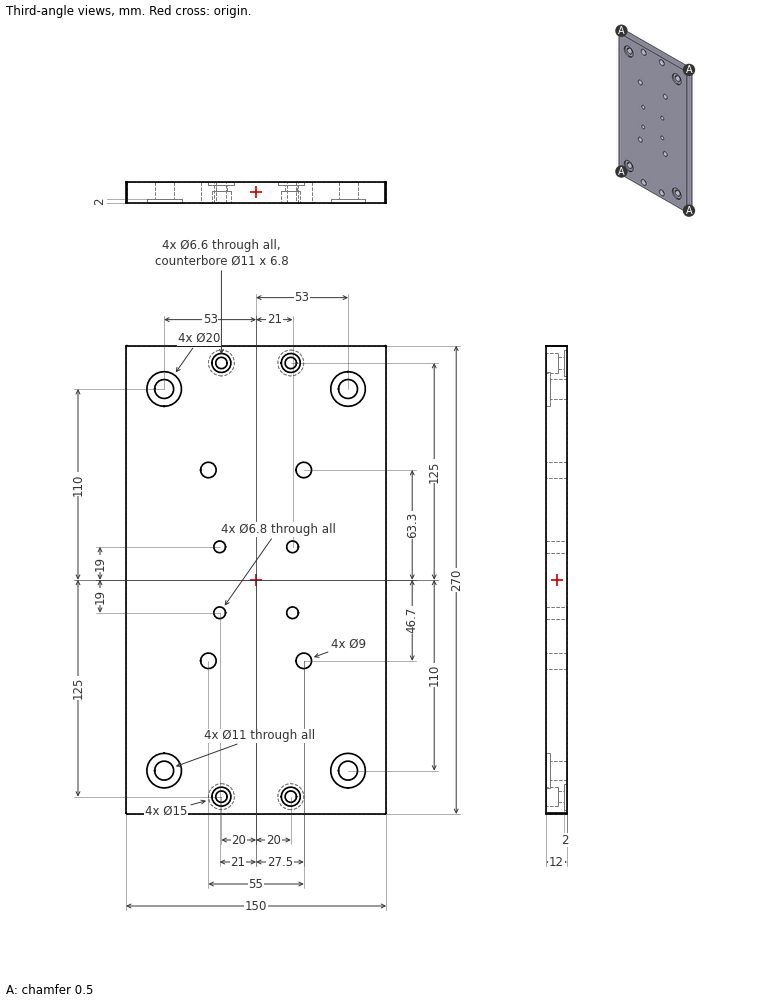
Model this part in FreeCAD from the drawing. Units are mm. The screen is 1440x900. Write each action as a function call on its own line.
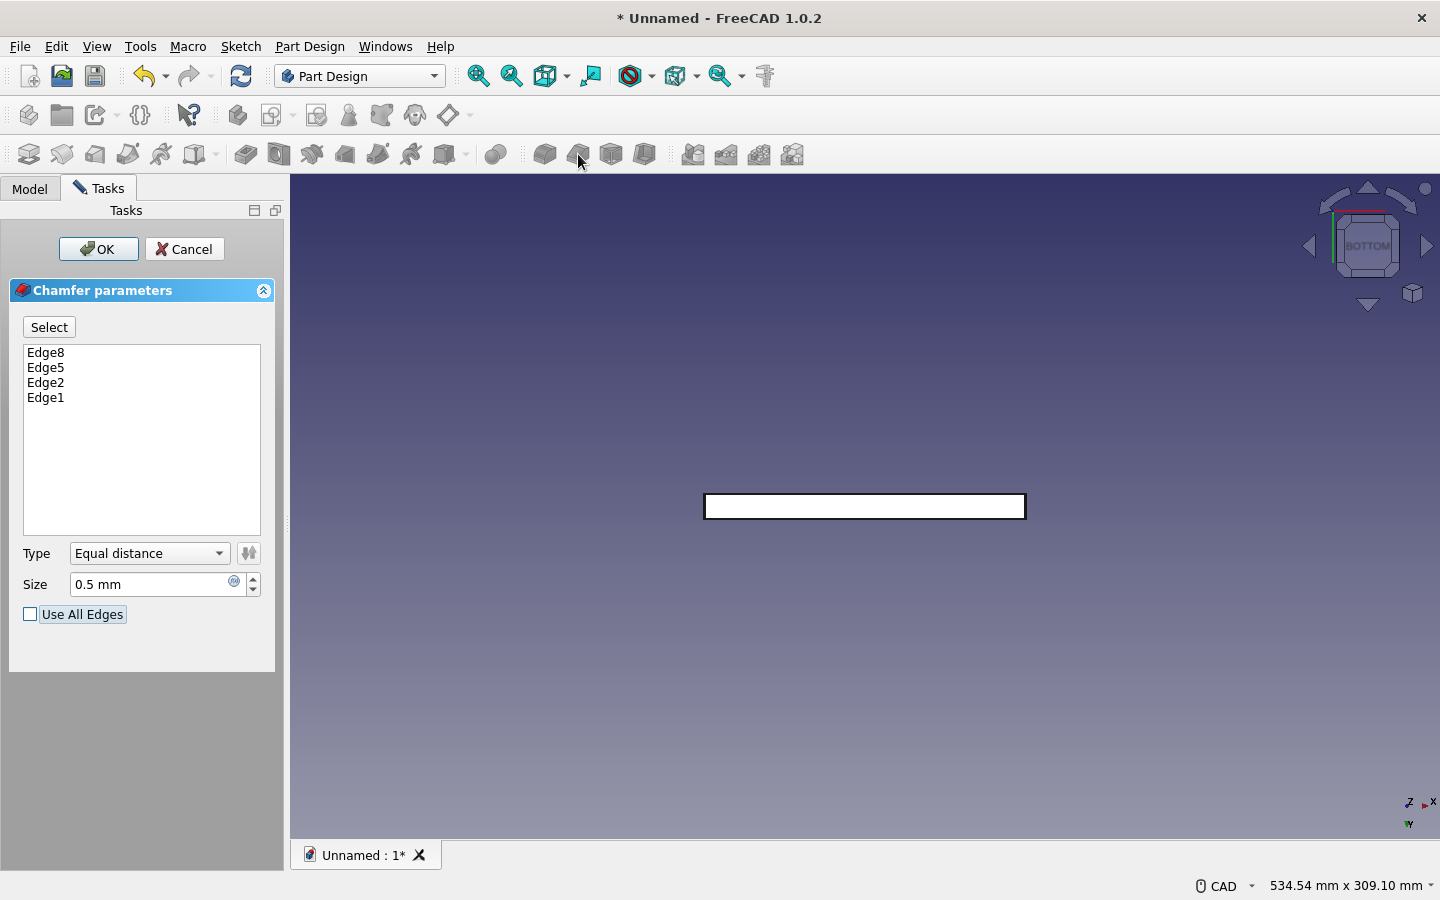
click(99, 249)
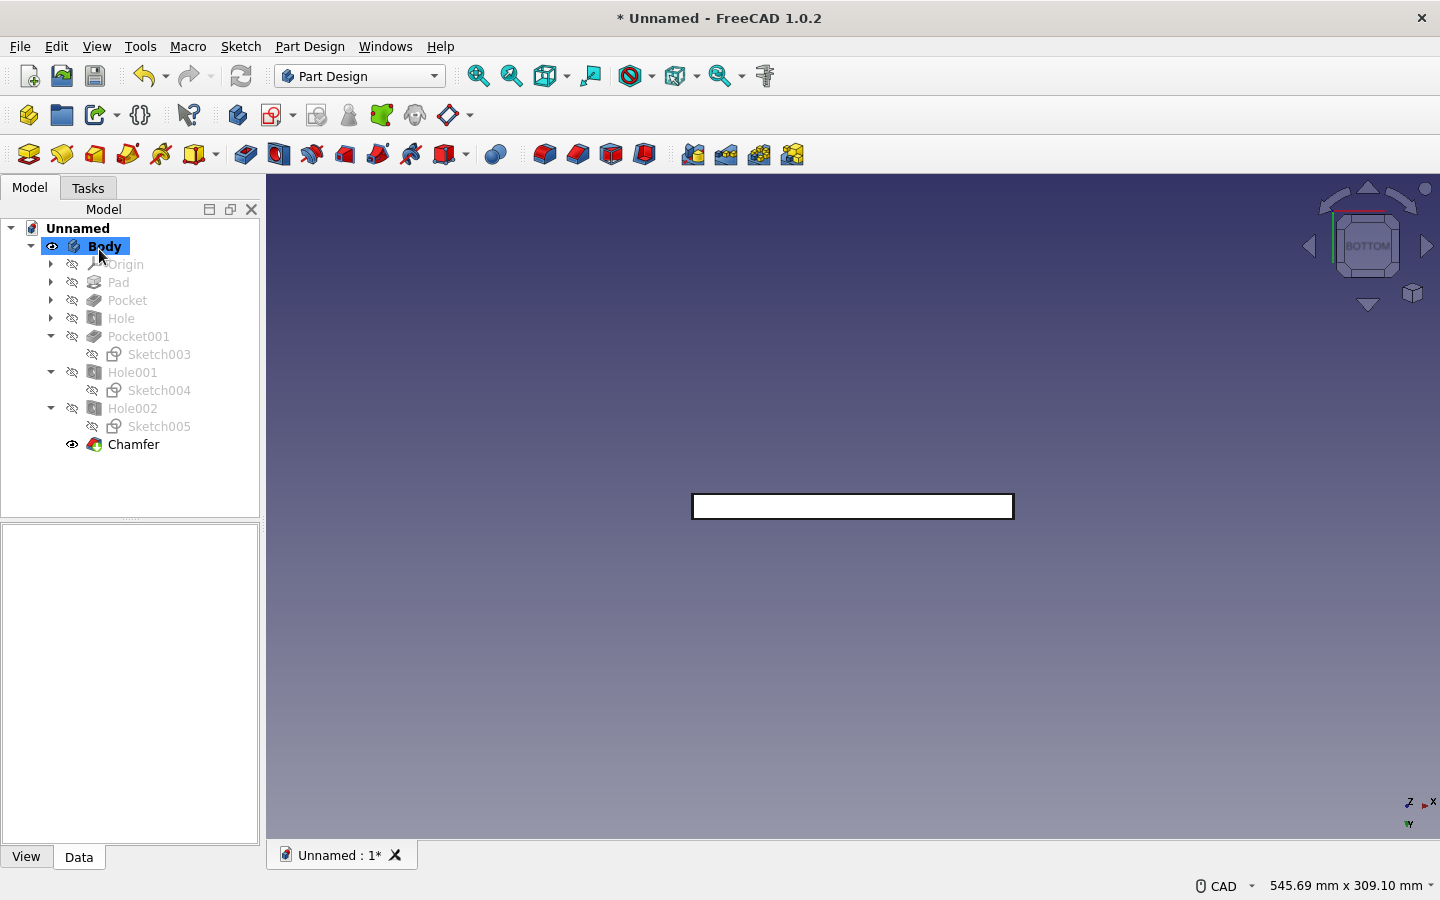
click(479, 76)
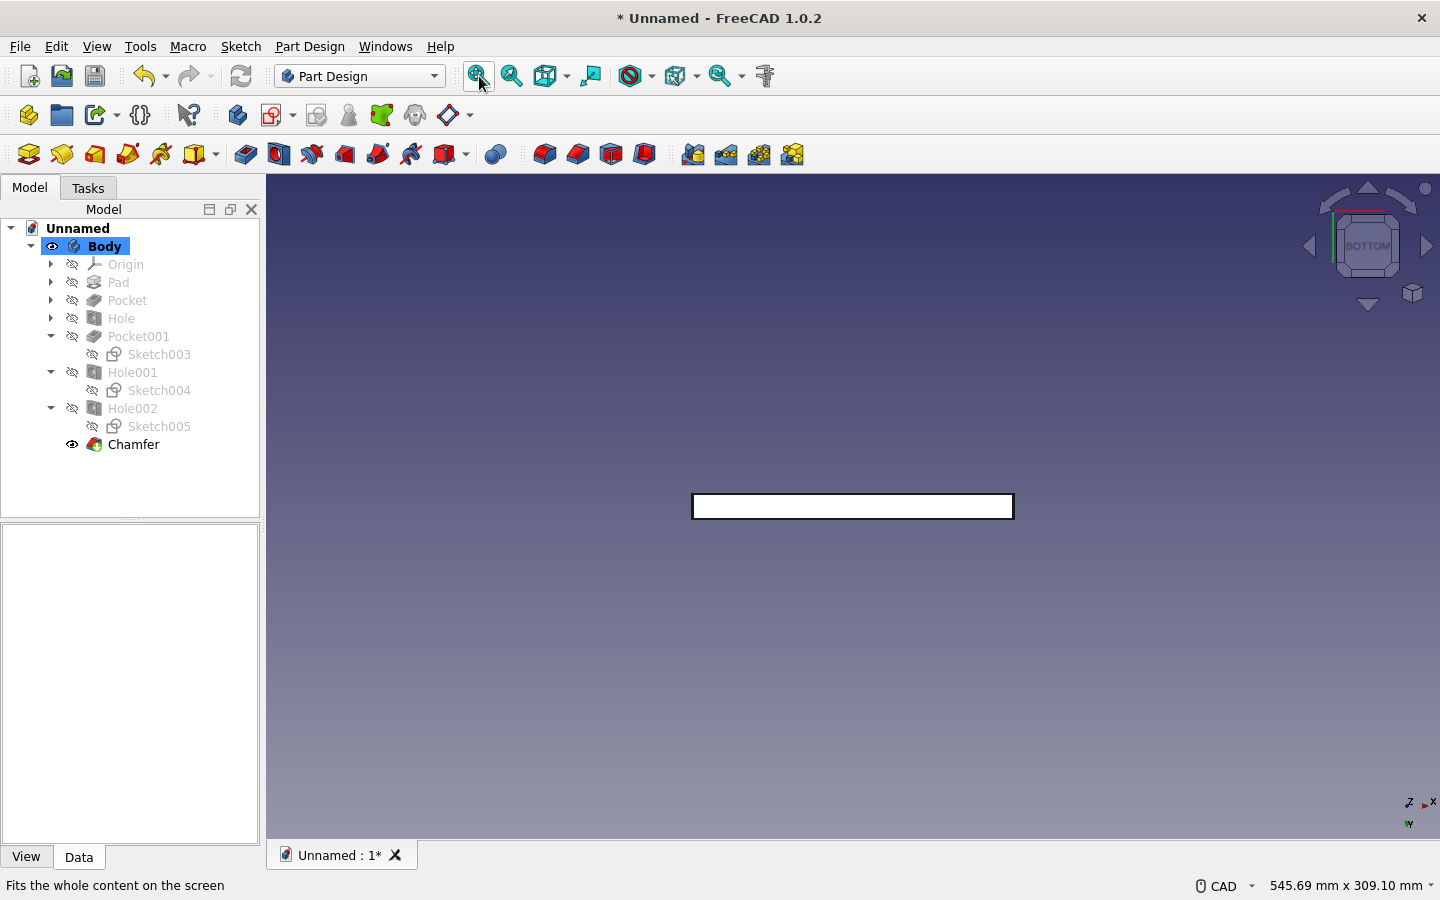
key(4)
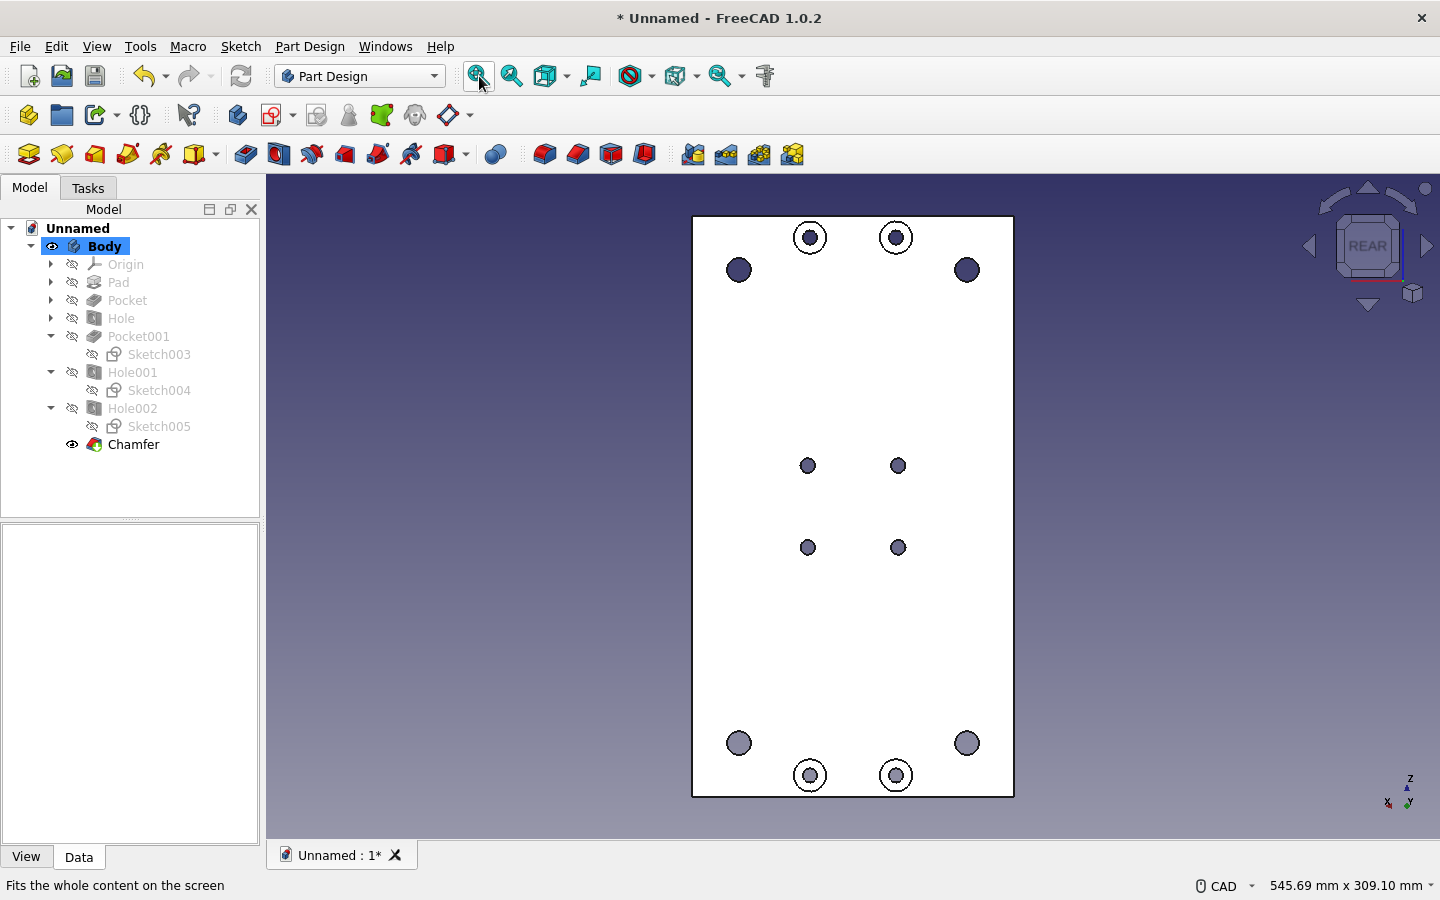
click(853, 340)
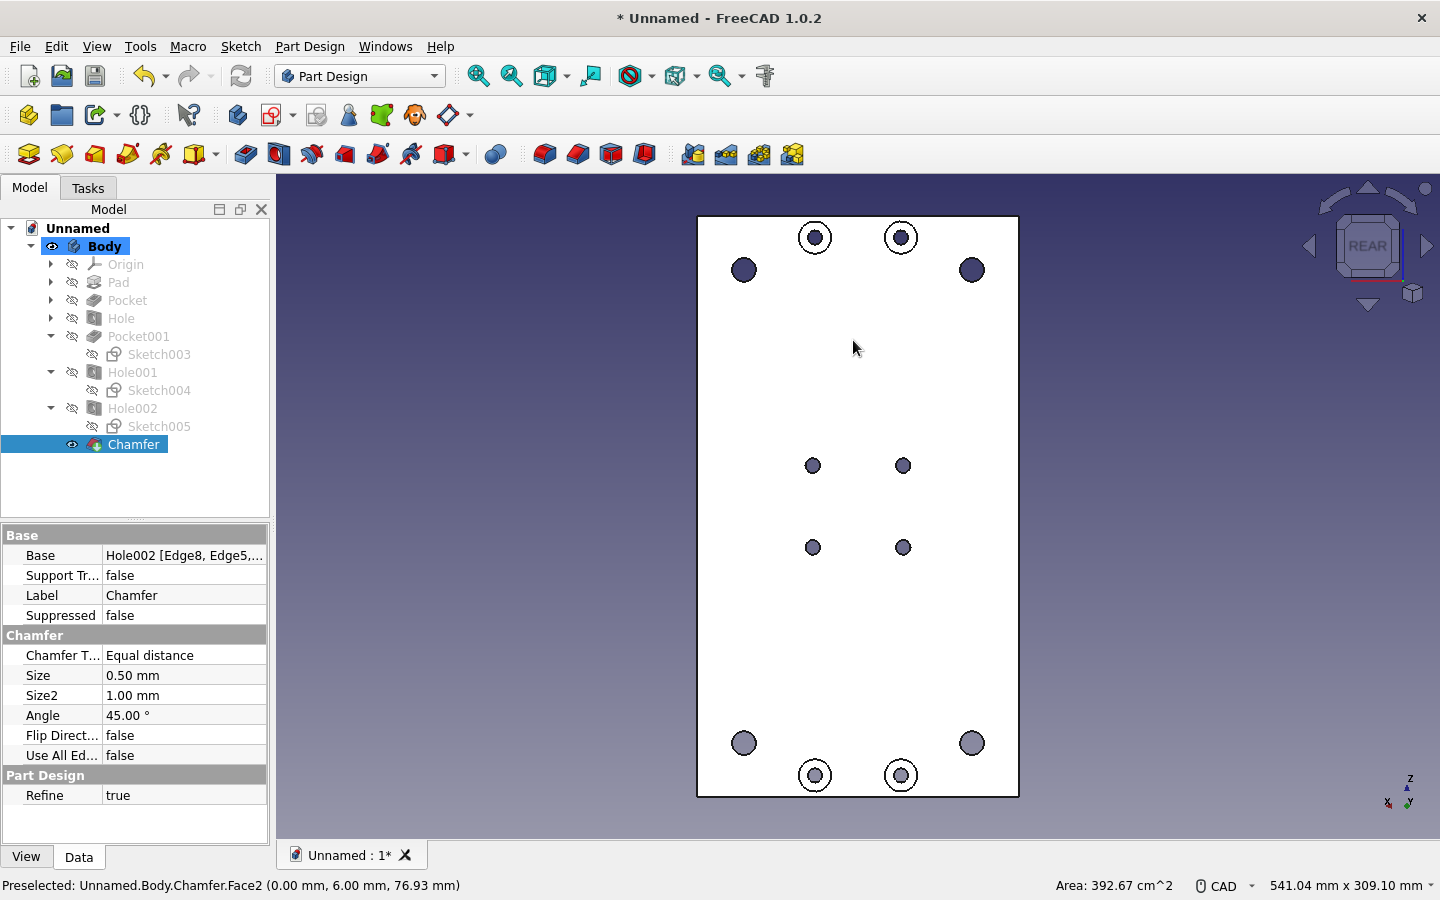
click(270, 116)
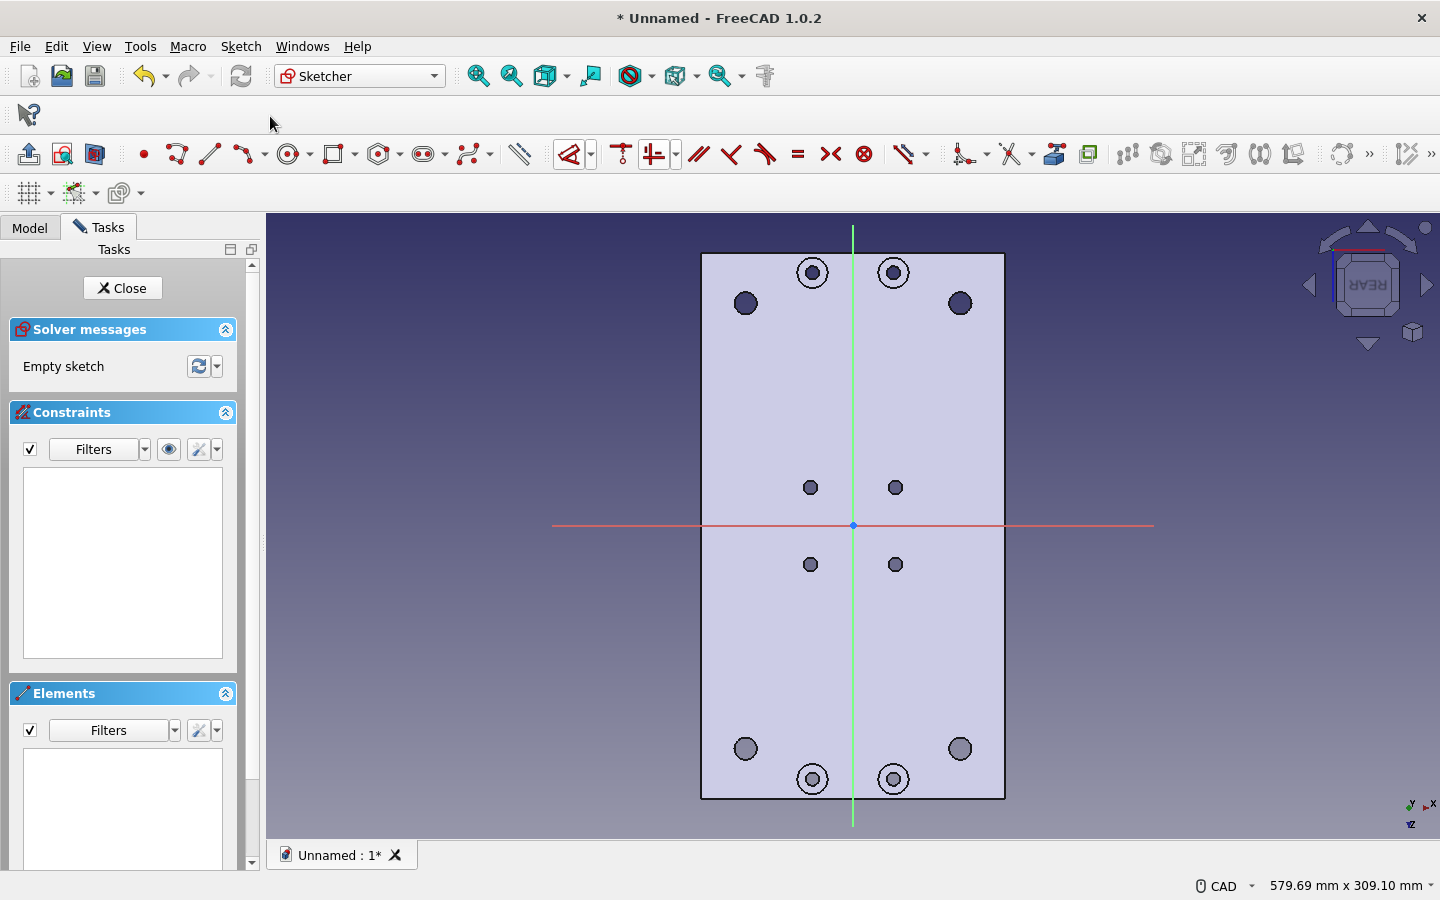
scroll(936, 563, up, 3)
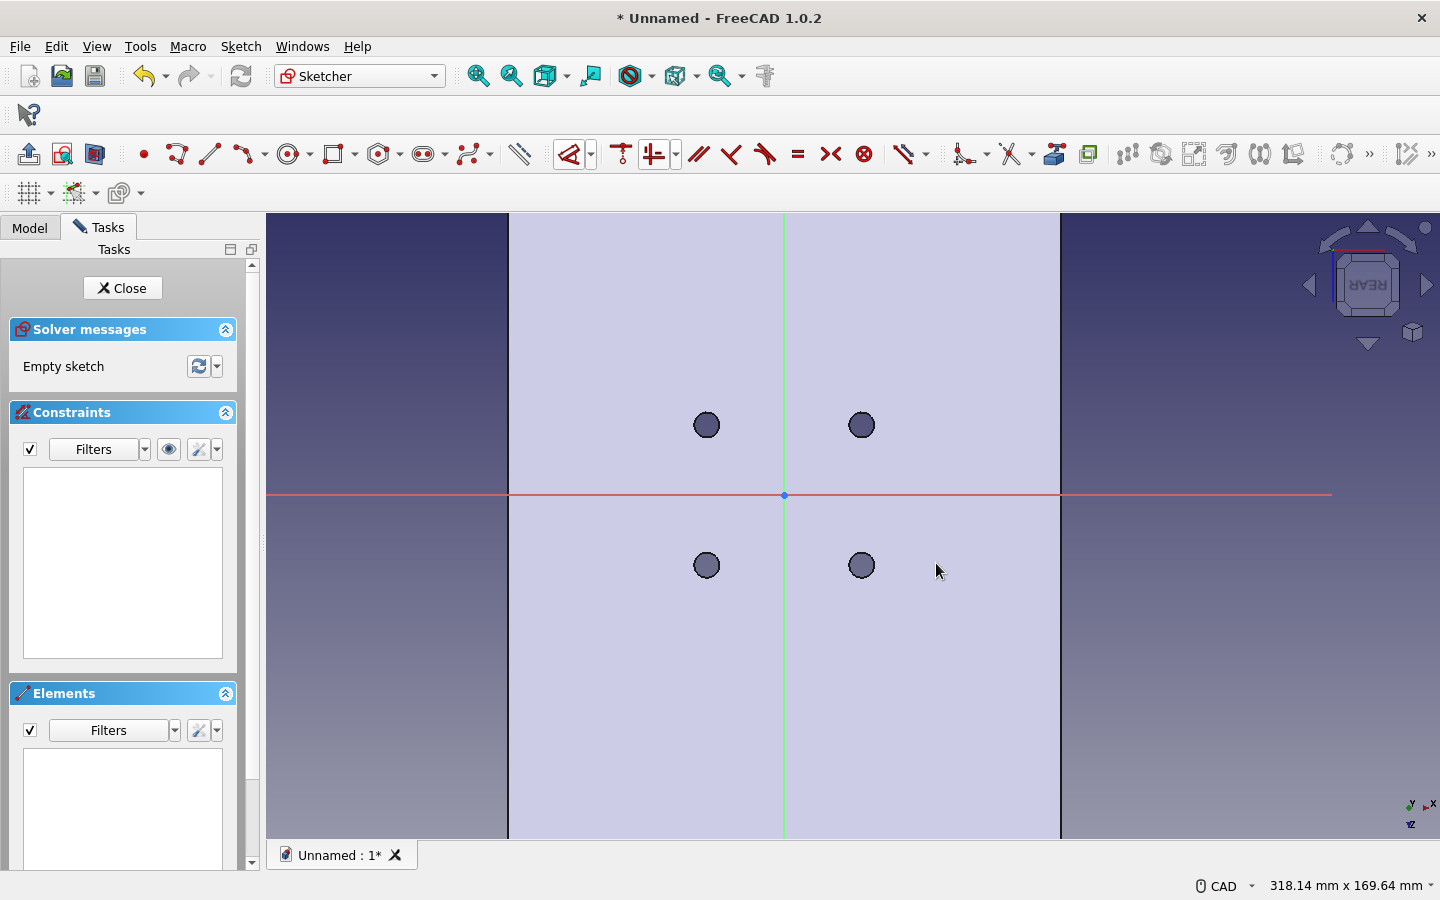
key(g)
key(c)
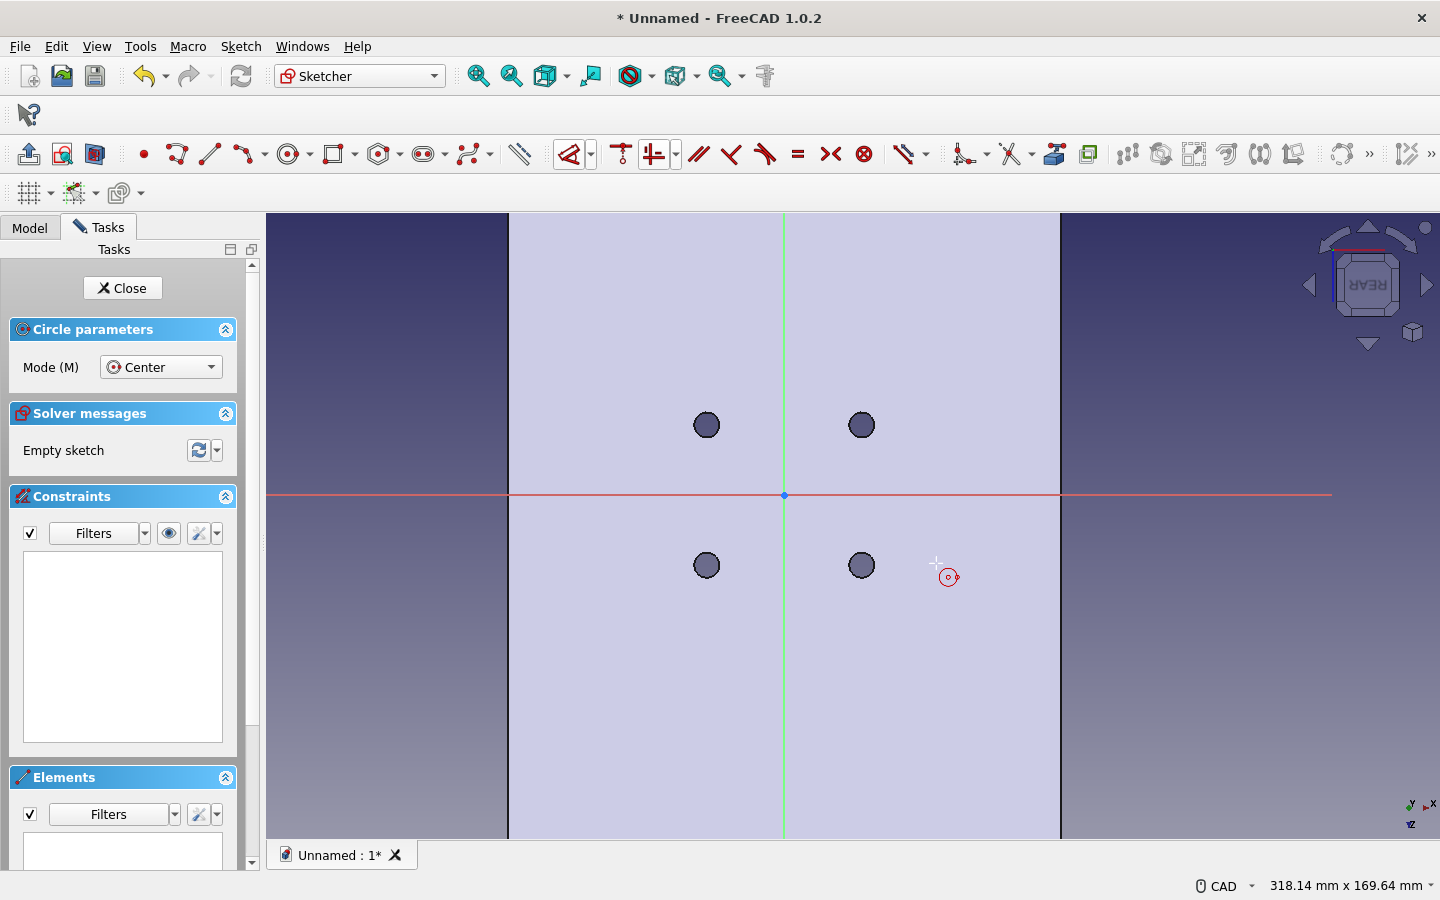
scroll(886, 323, up, 2)